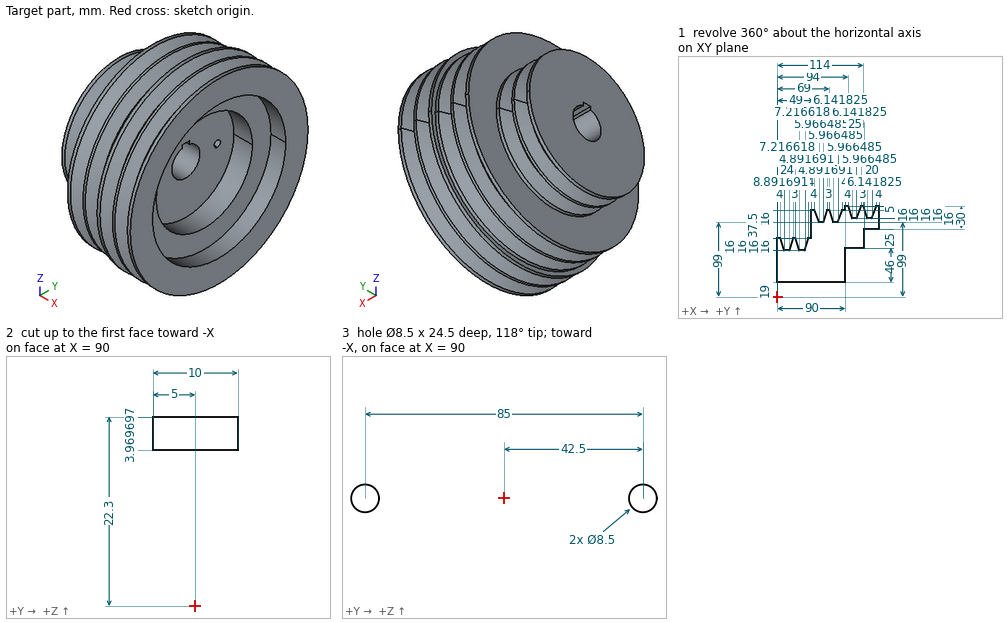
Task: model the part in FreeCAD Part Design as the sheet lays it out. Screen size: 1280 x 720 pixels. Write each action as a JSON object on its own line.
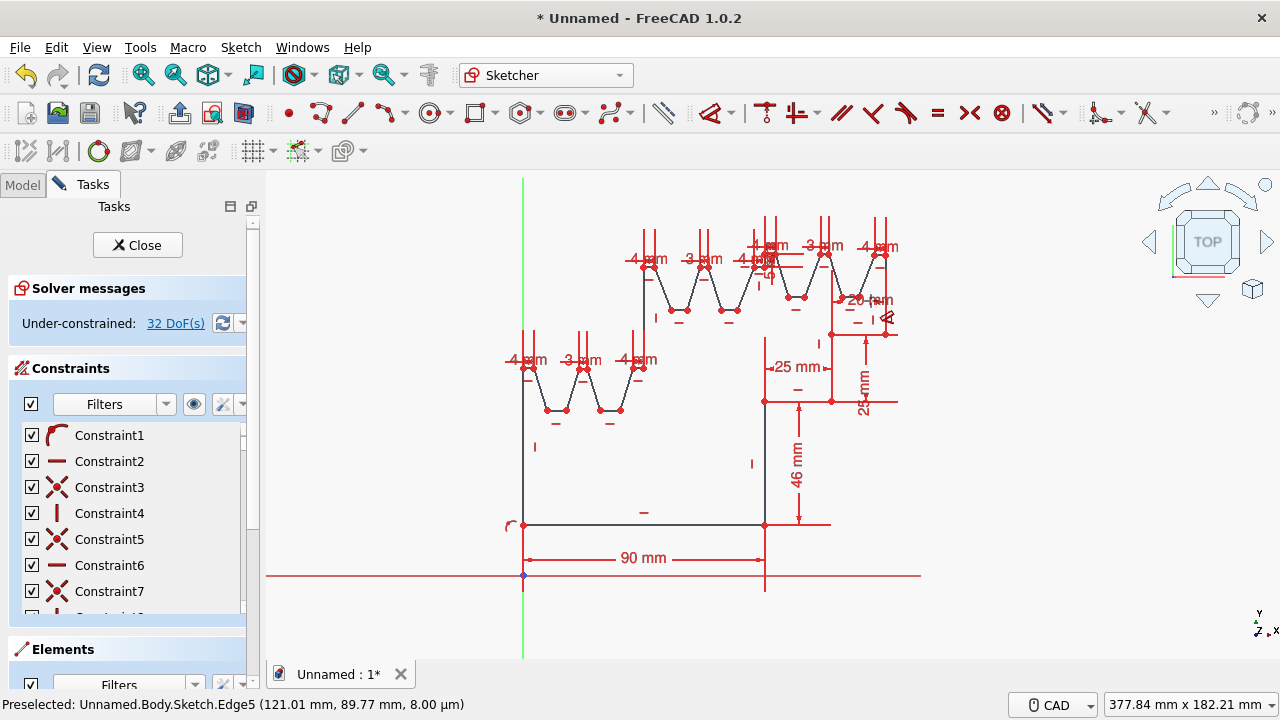
{"action": "left_click", "coordinate": [886, 311]}
{"action": "left_click", "coordinate": [920, 277]}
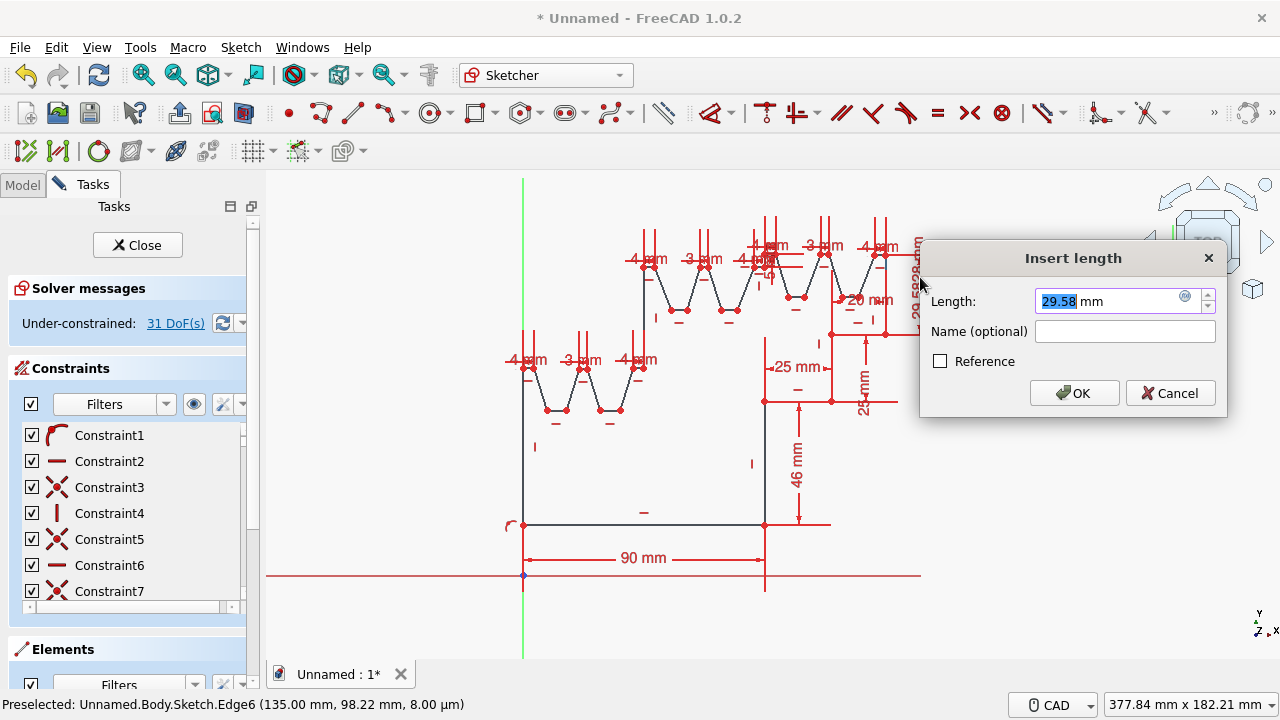
{"action": "type", "text": "30"}
{"action": "key", "text": "Return"}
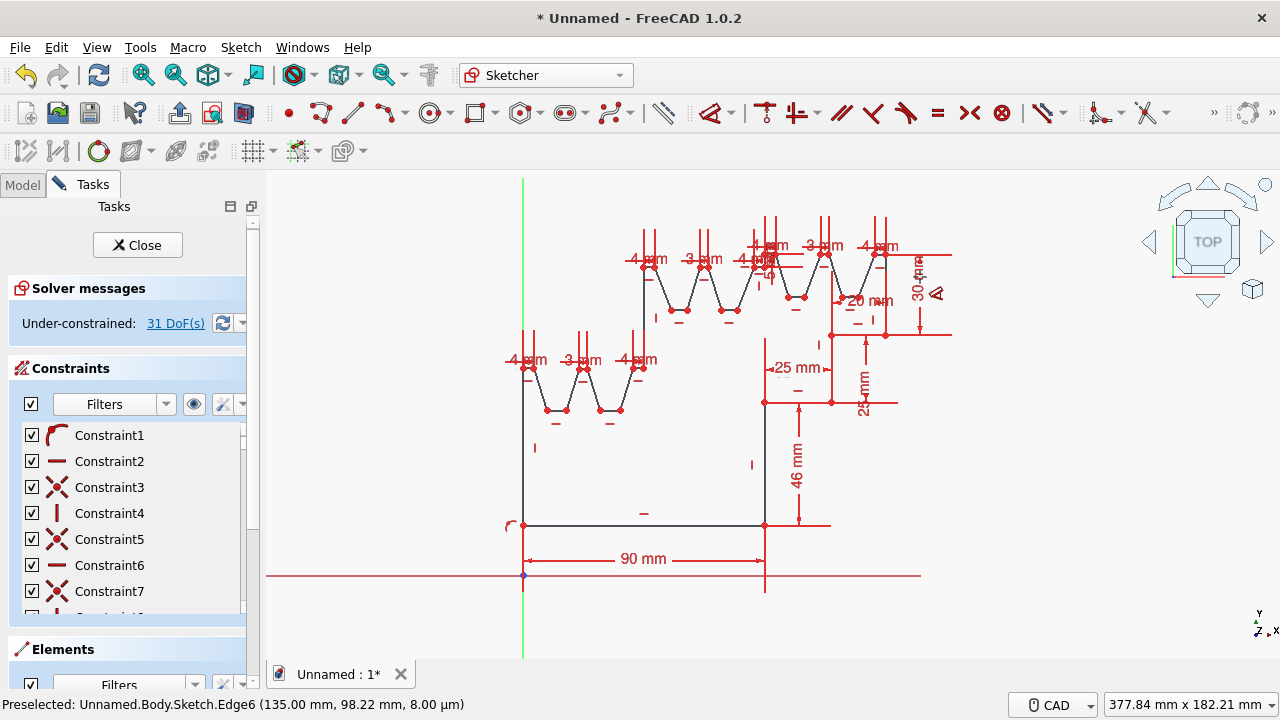
{"action": "left_click", "coordinate": [523, 526]}
{"action": "left_click", "coordinate": [489, 551]}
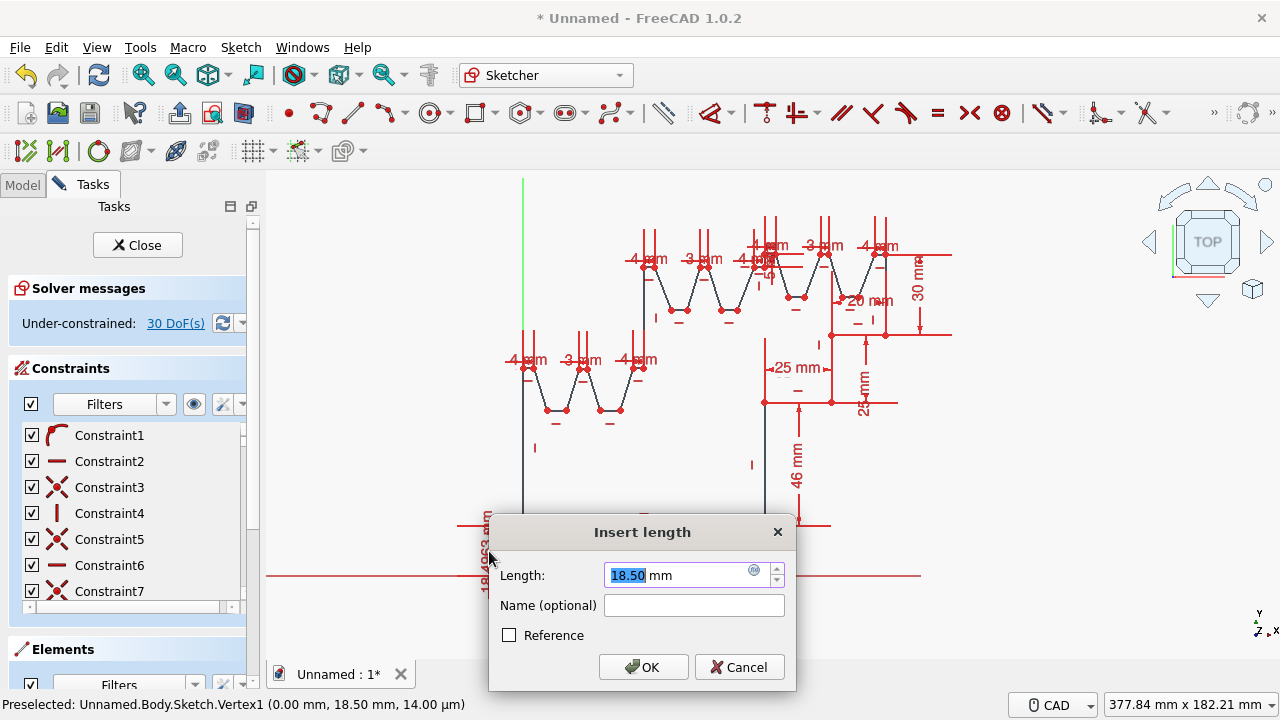
{"action": "type", "text": "19"}
{"action": "key", "text": "Return"}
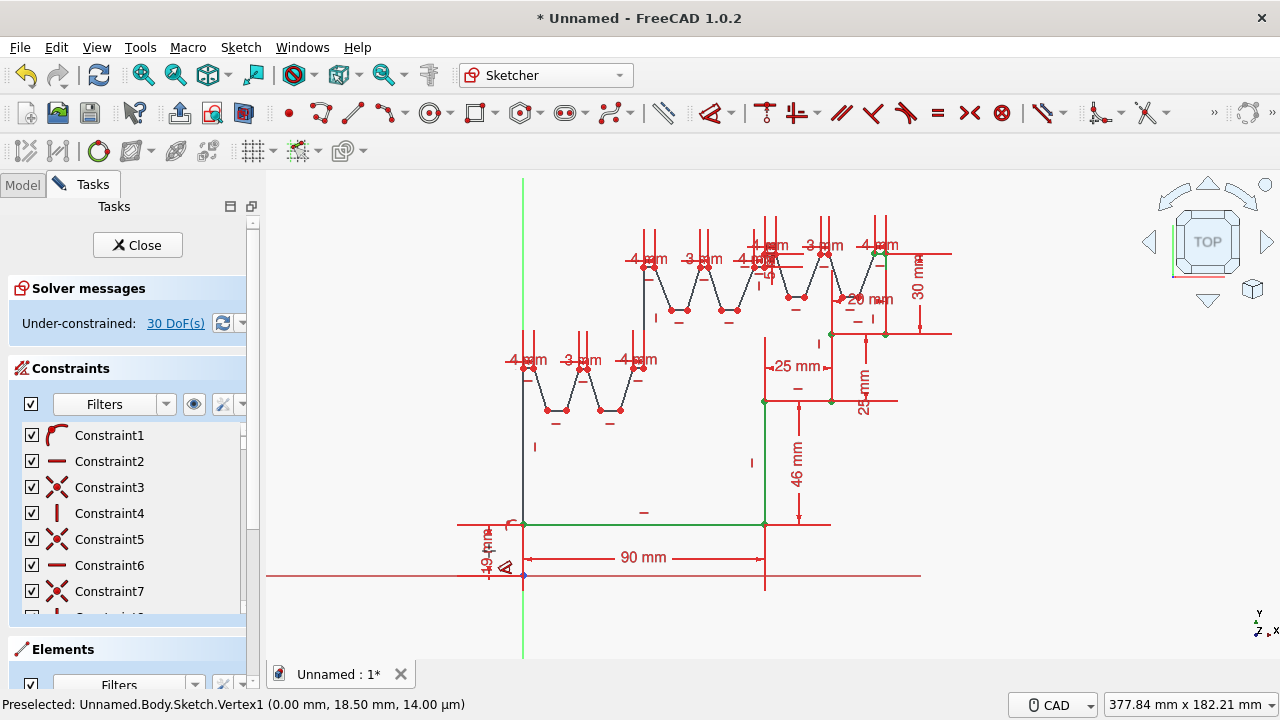
{"action": "left_click", "coordinate": [776, 254]}
{"action": "left_click", "coordinate": [649, 610]}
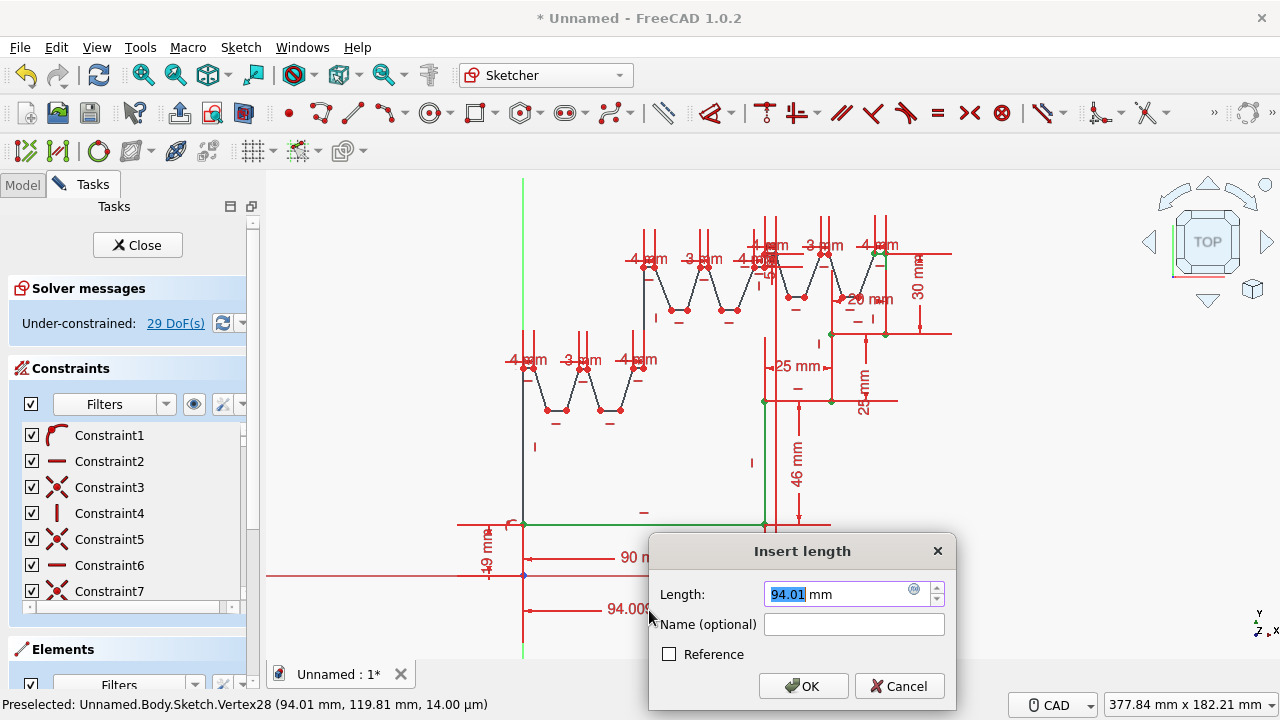
{"action": "type", "text": "94"}
{"action": "key", "text": "Return"}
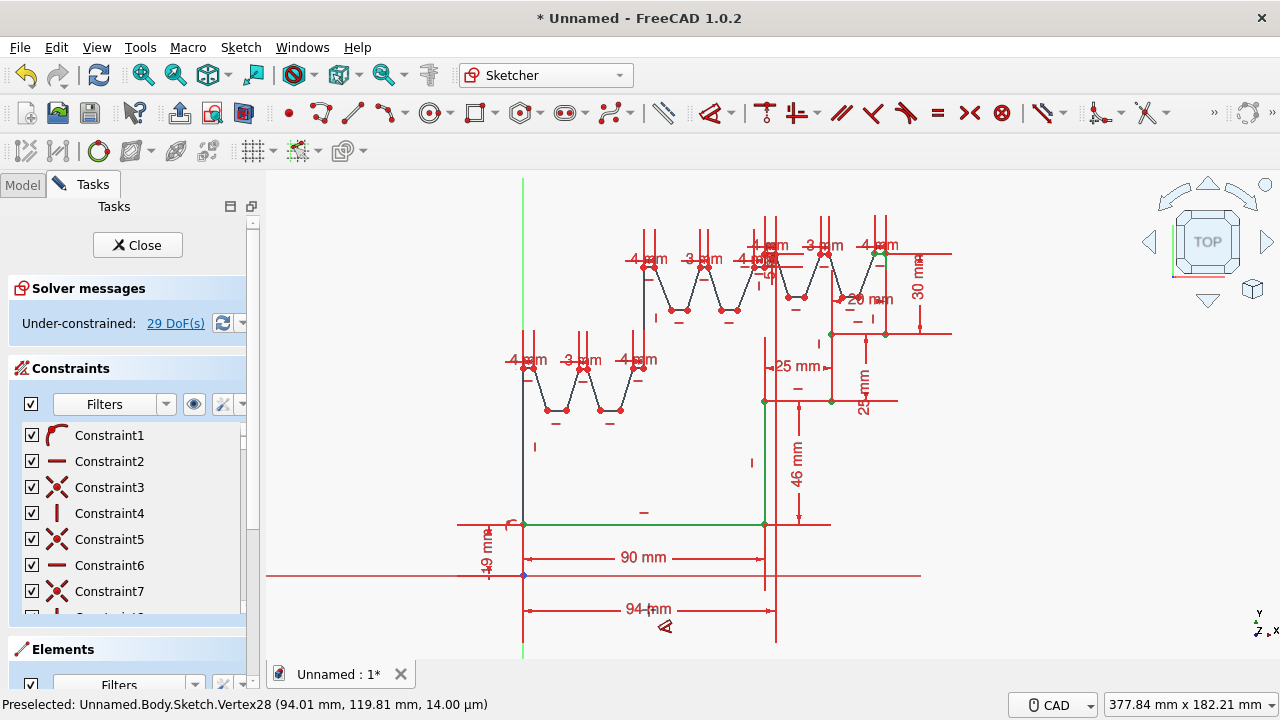
{"action": "left_click", "coordinate": [737, 310]}
{"action": "left_click", "coordinate": [489, 443]}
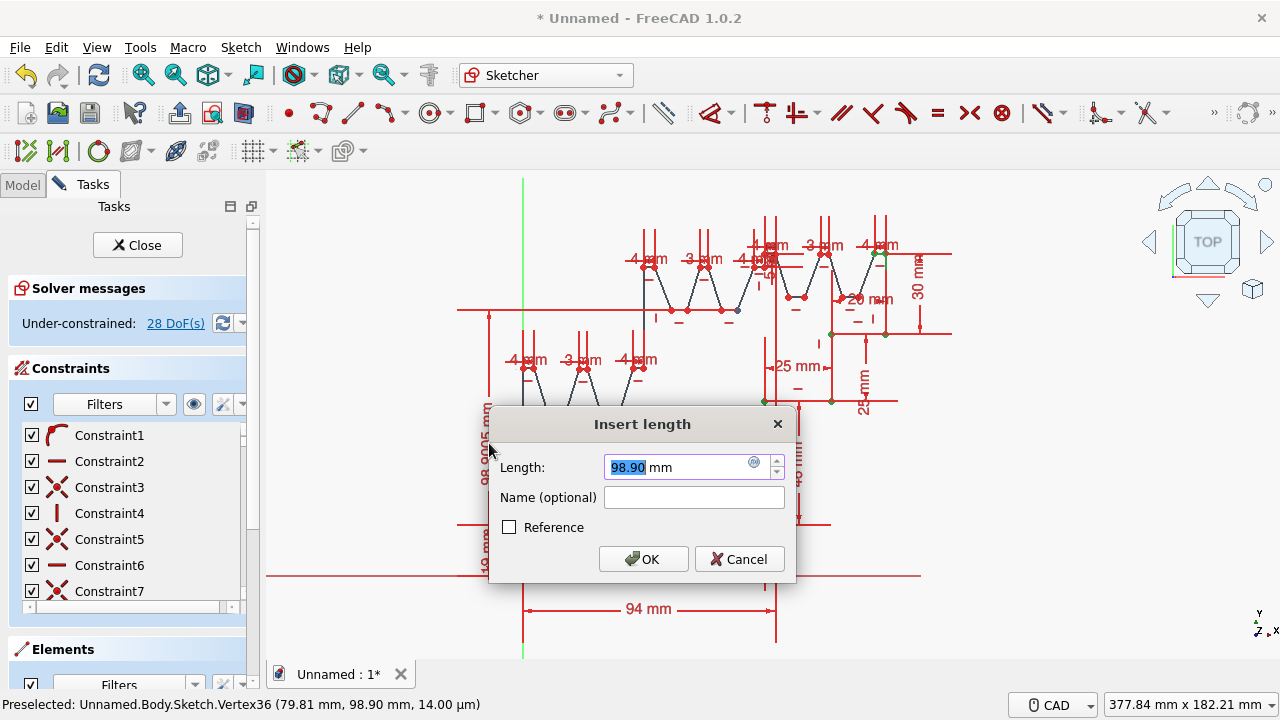
{"action": "type", "text": "99"}
{"action": "key", "text": "Return"}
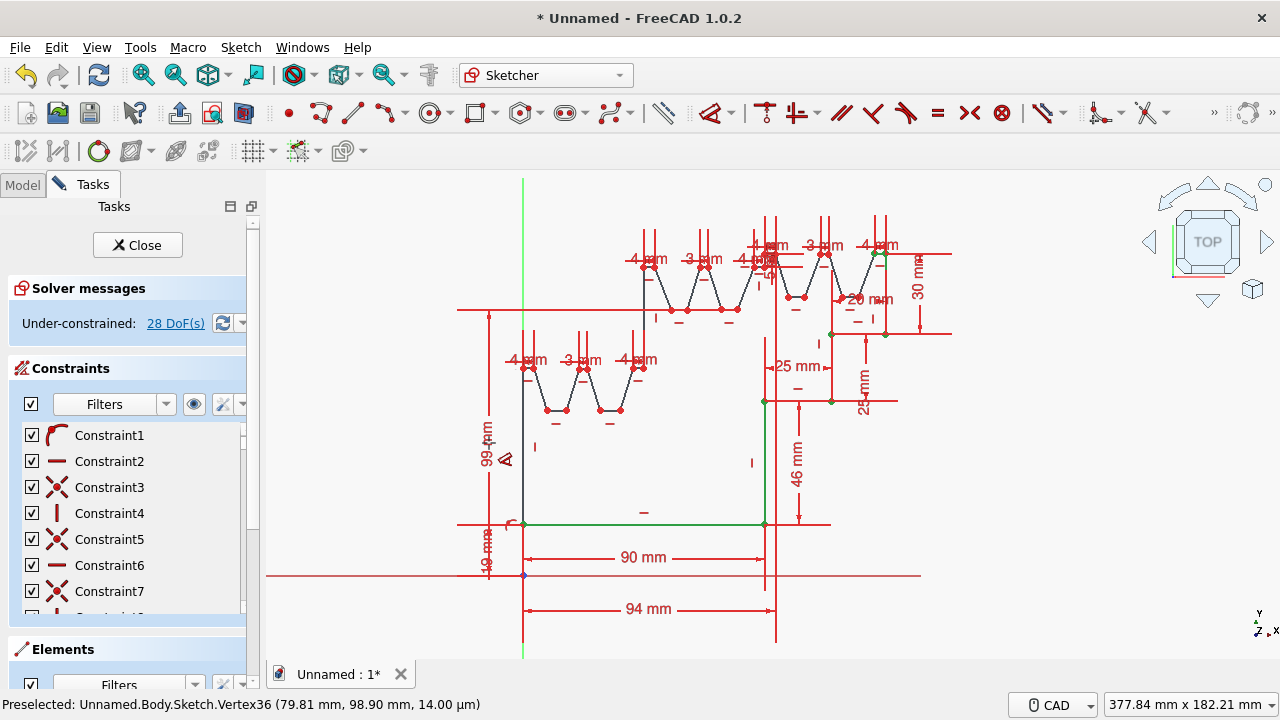
{"action": "scroll", "coordinate": [708, 267], "scroll_direction": "up", "scroll_amount": 3}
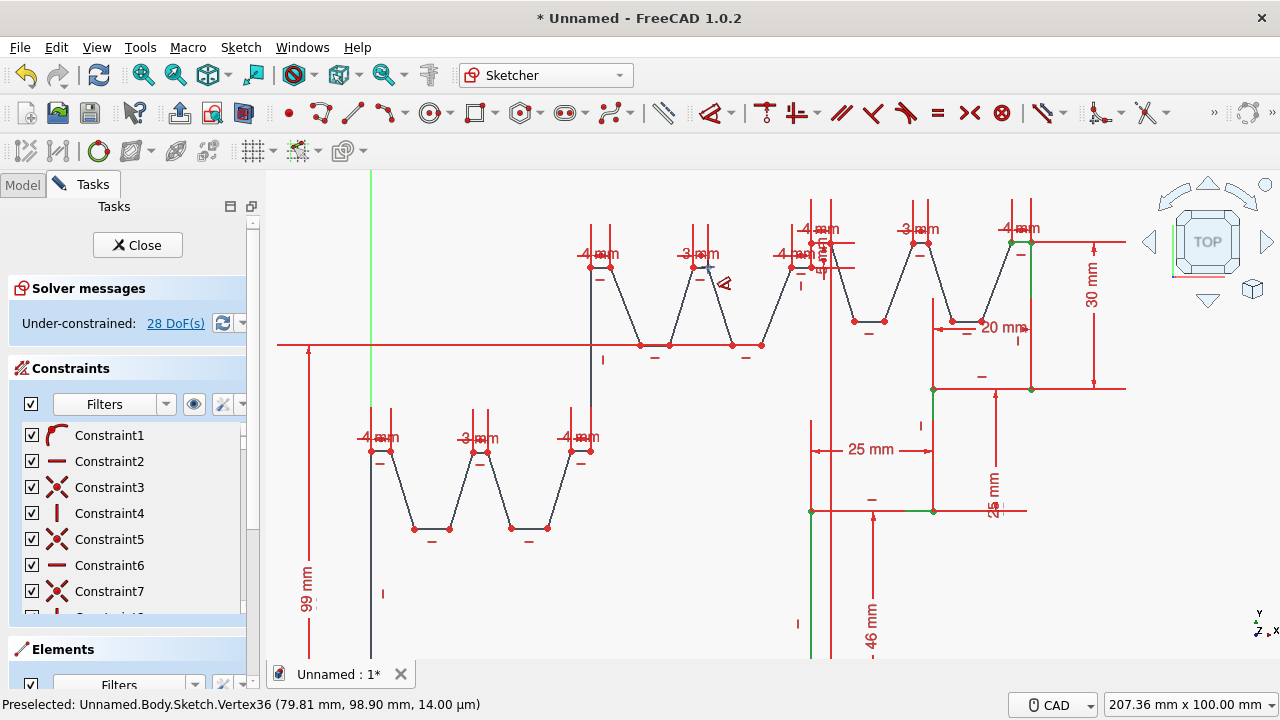
{"action": "left_click", "coordinate": [708, 268]}
{"action": "left_click", "coordinate": [540, 234]}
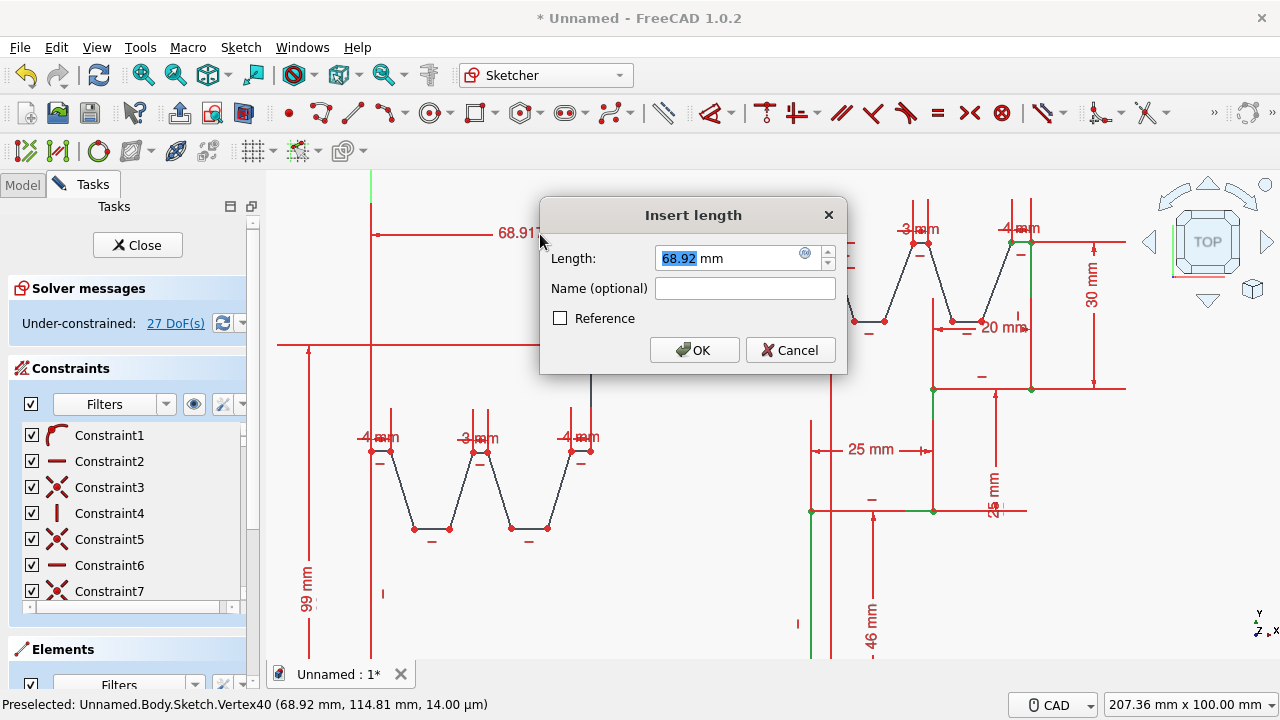
{"action": "type", "text": "69"}
{"action": "key", "text": "Return"}